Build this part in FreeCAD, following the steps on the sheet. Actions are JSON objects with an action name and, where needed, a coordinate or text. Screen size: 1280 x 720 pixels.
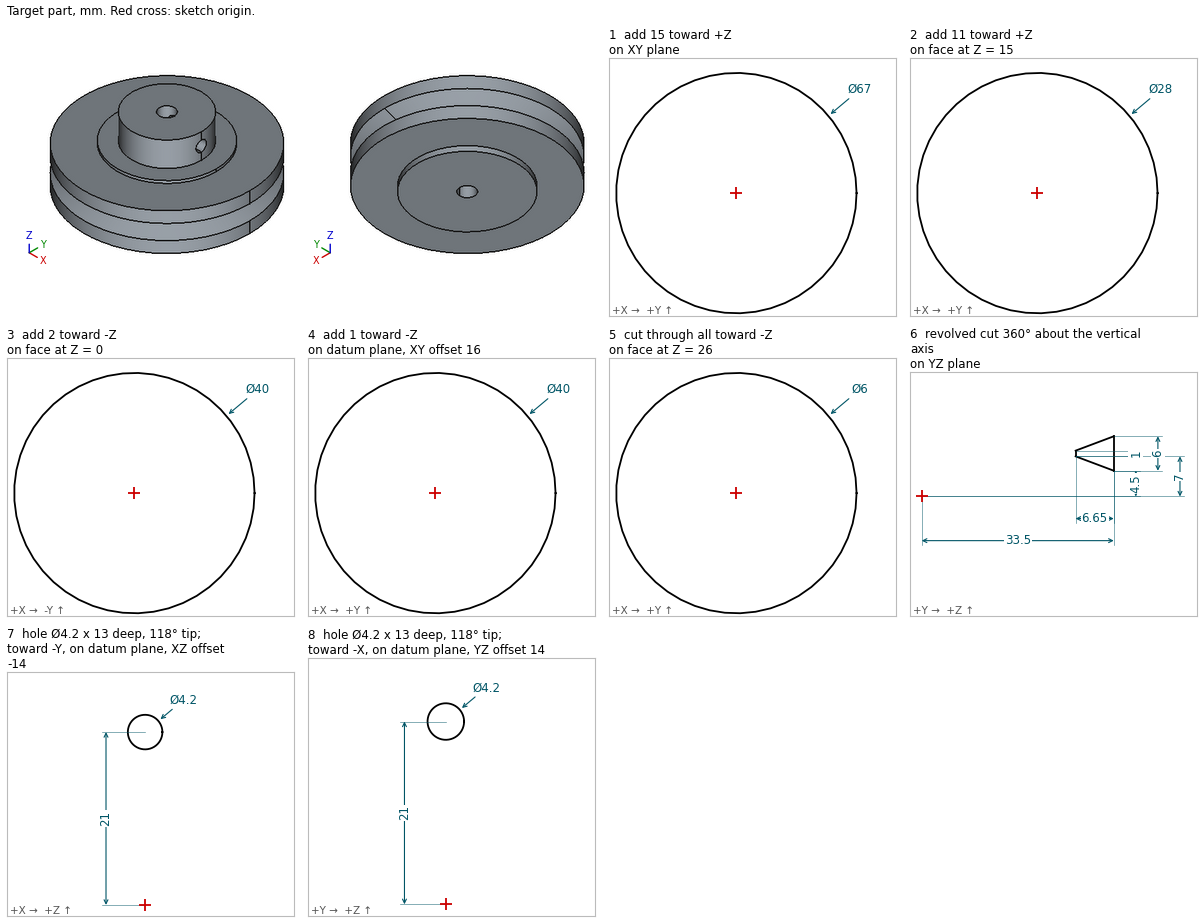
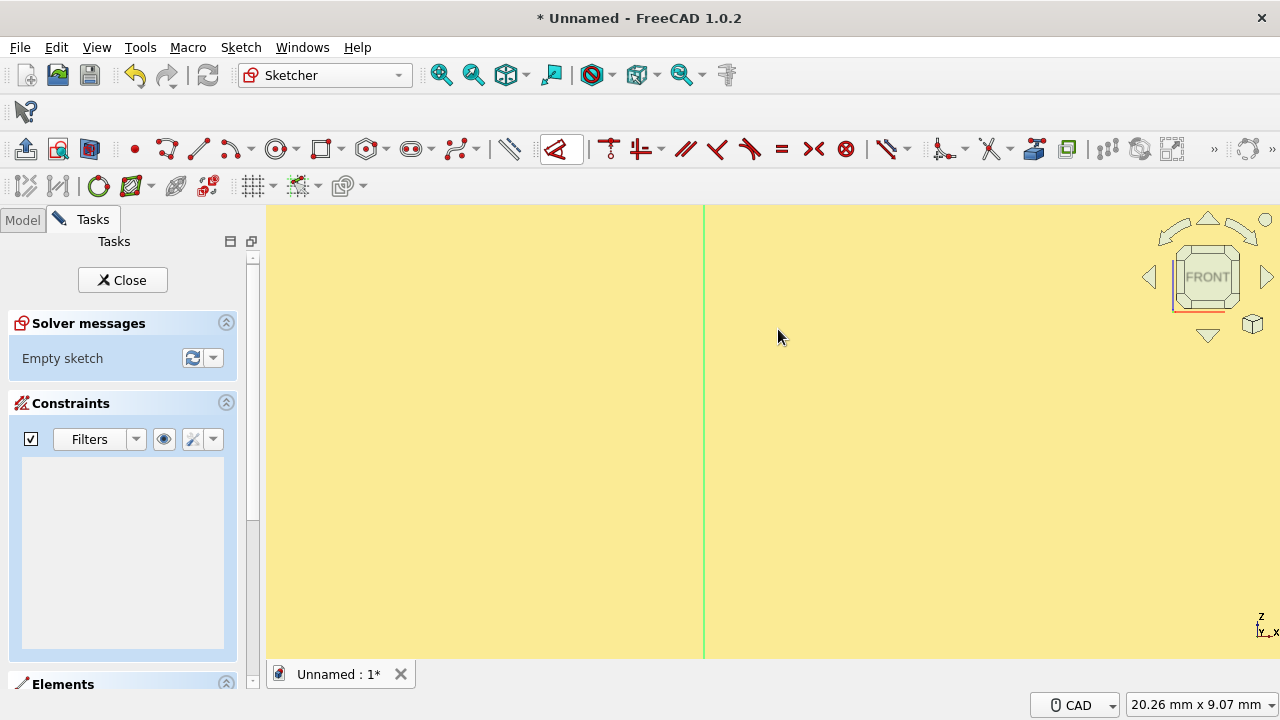
{"action": "left_click", "coordinate": [276, 150]}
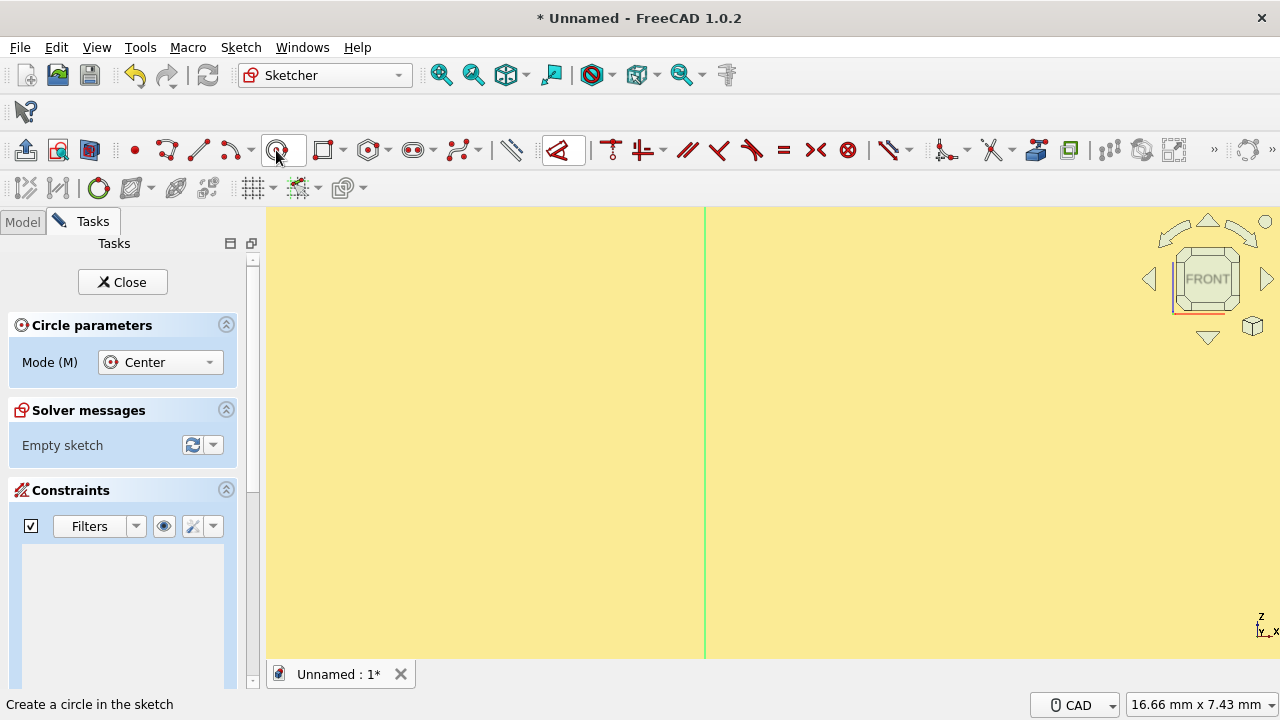
{"action": "left_click", "coordinate": [705, 430]}
{"action": "left_click", "coordinate": [795, 339]}
{"action": "key", "text": "Escape"}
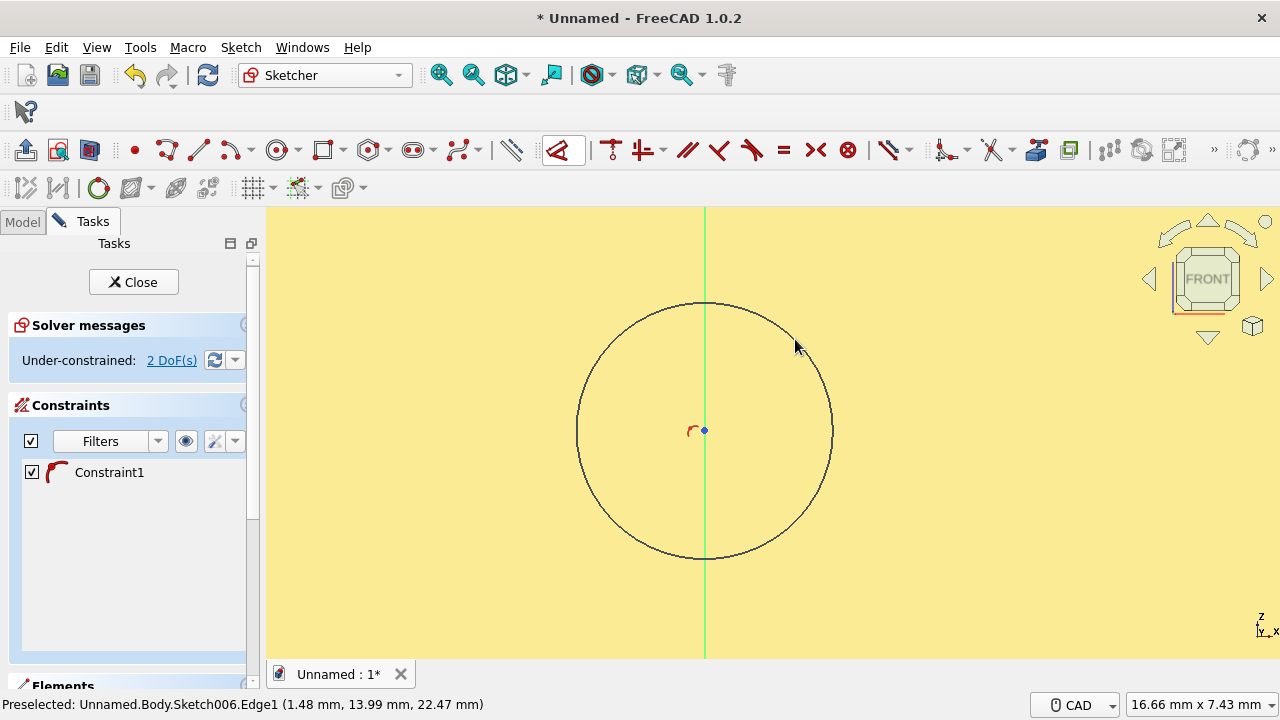
{"action": "left_click", "coordinate": [795, 340]}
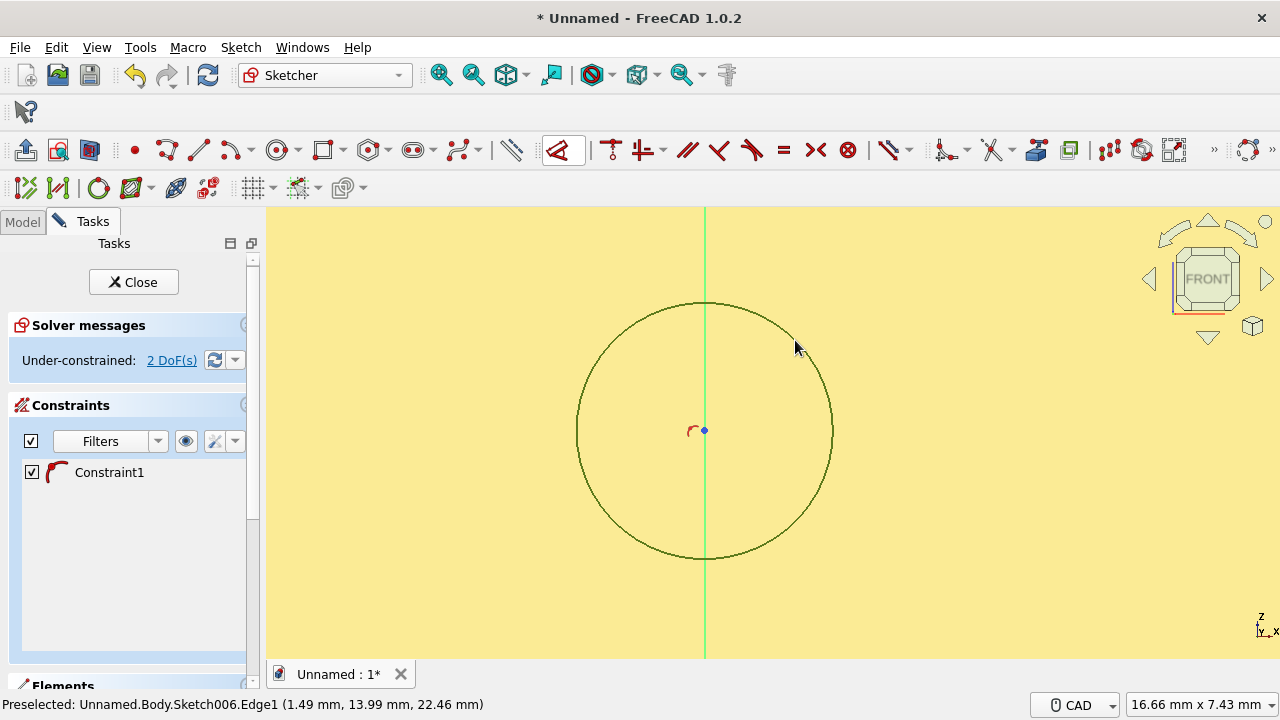
{"action": "key", "text": "k o"}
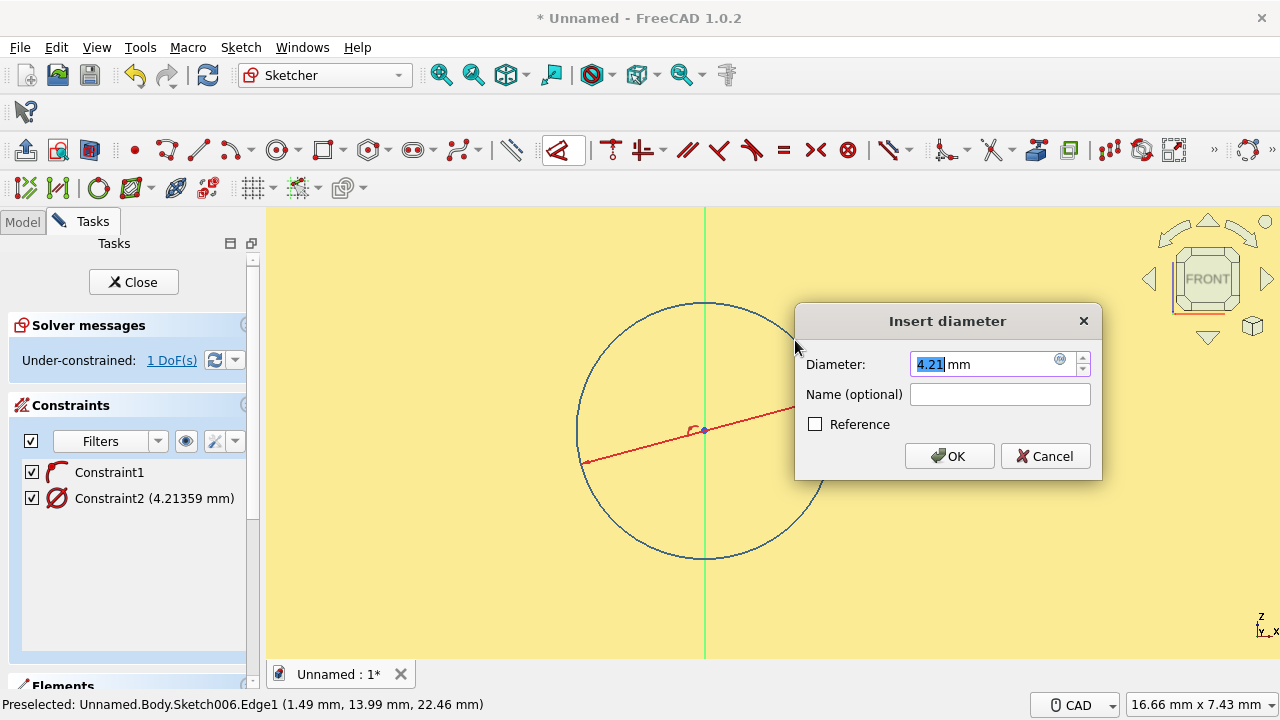
{"action": "type", "text": "4.2"}
{"action": "key", "text": "Return"}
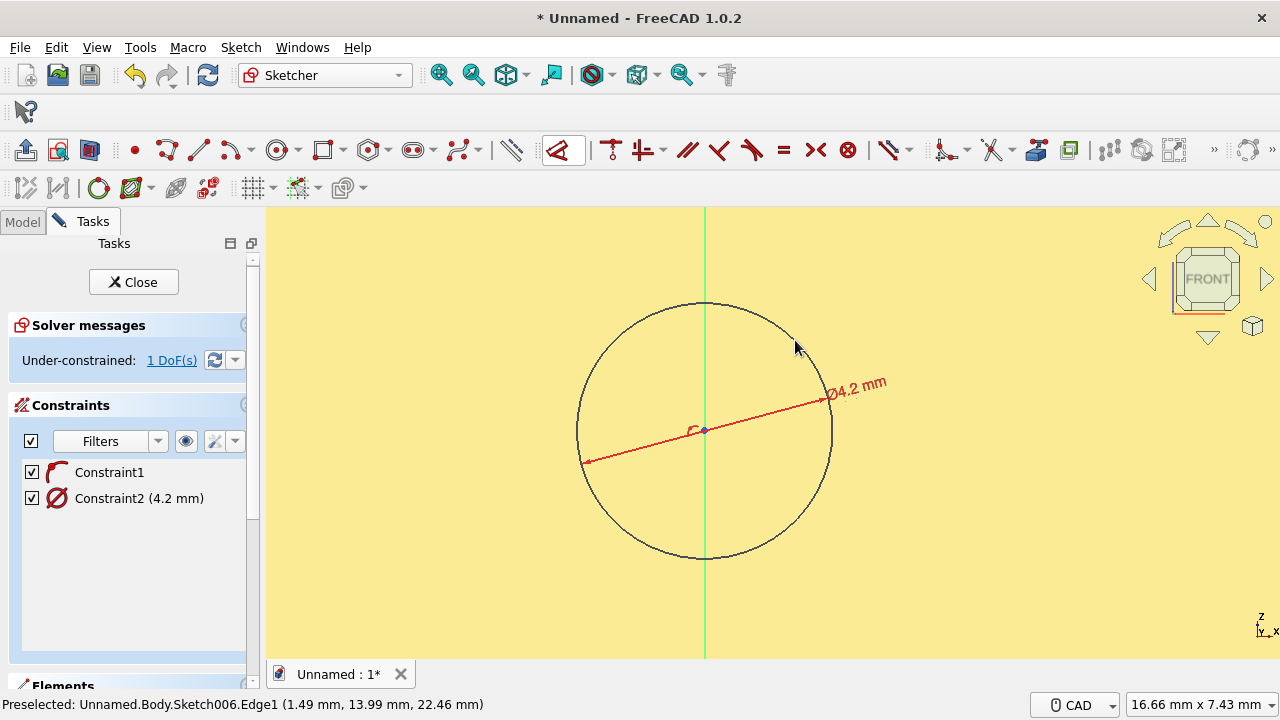
{"action": "left_click", "coordinate": [705, 431]}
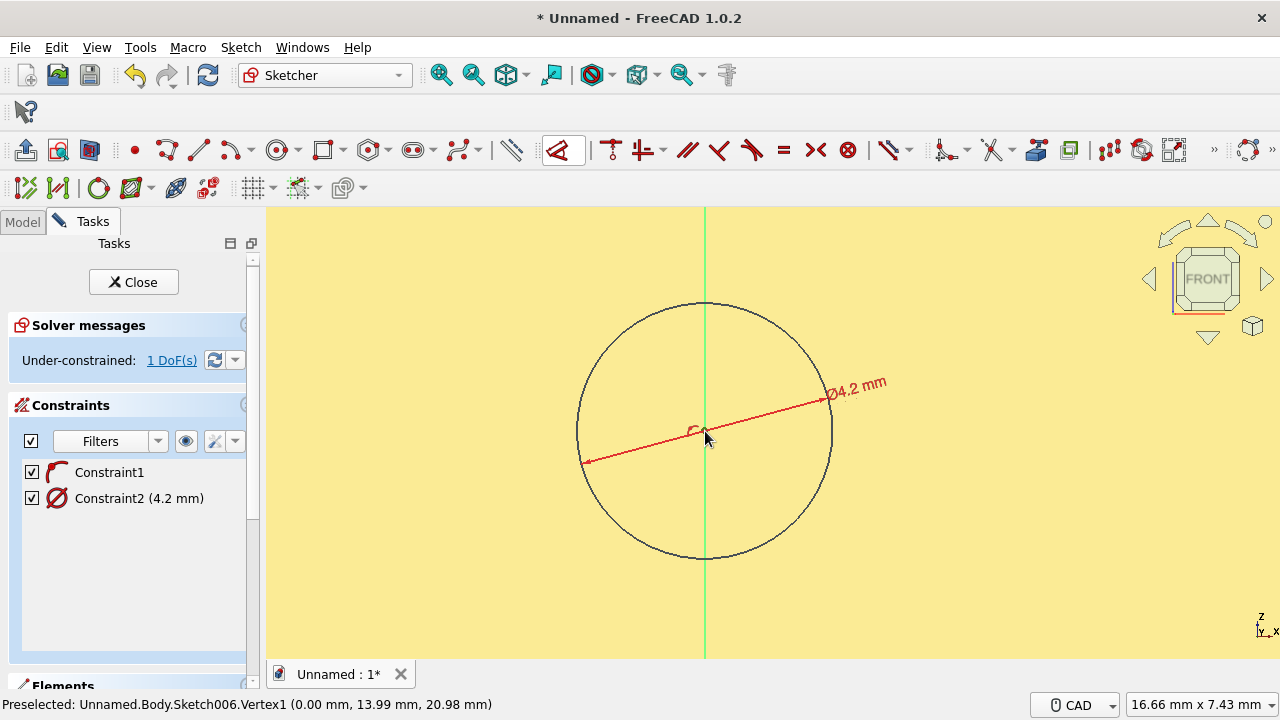
{"action": "key", "text": "i"}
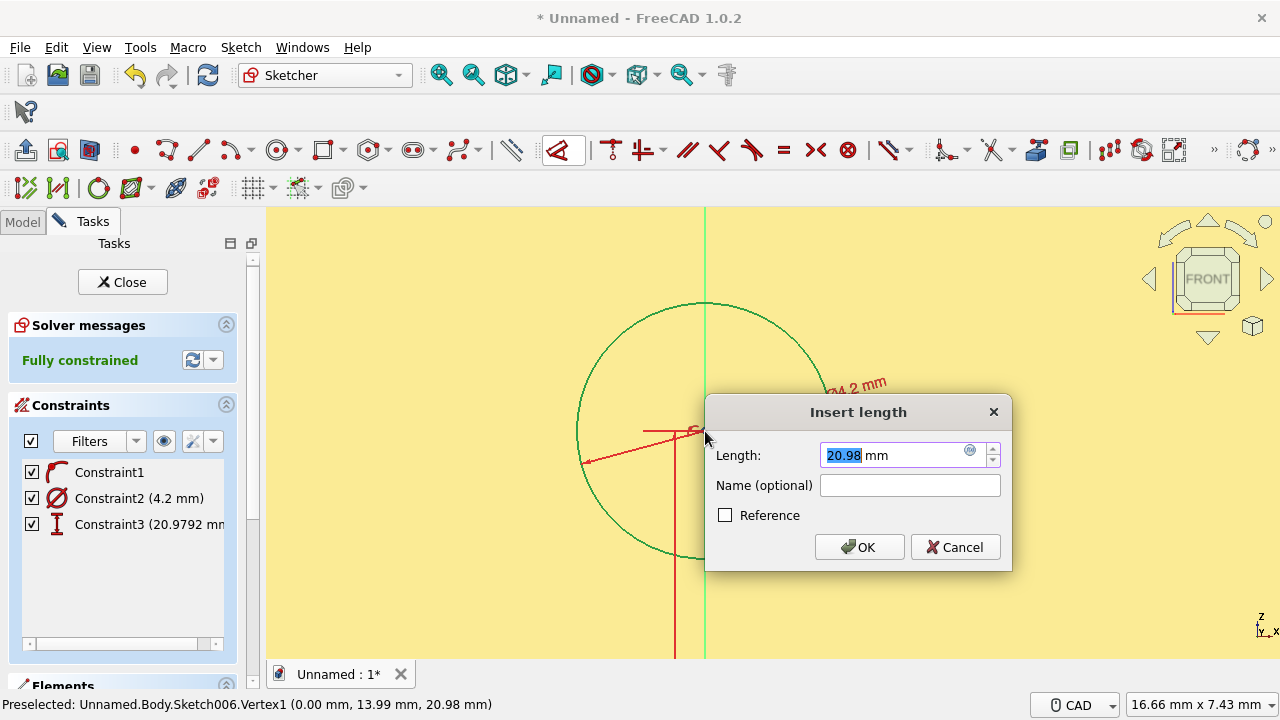
{"action": "type", "text": "21"}
{"action": "key", "text": "Return"}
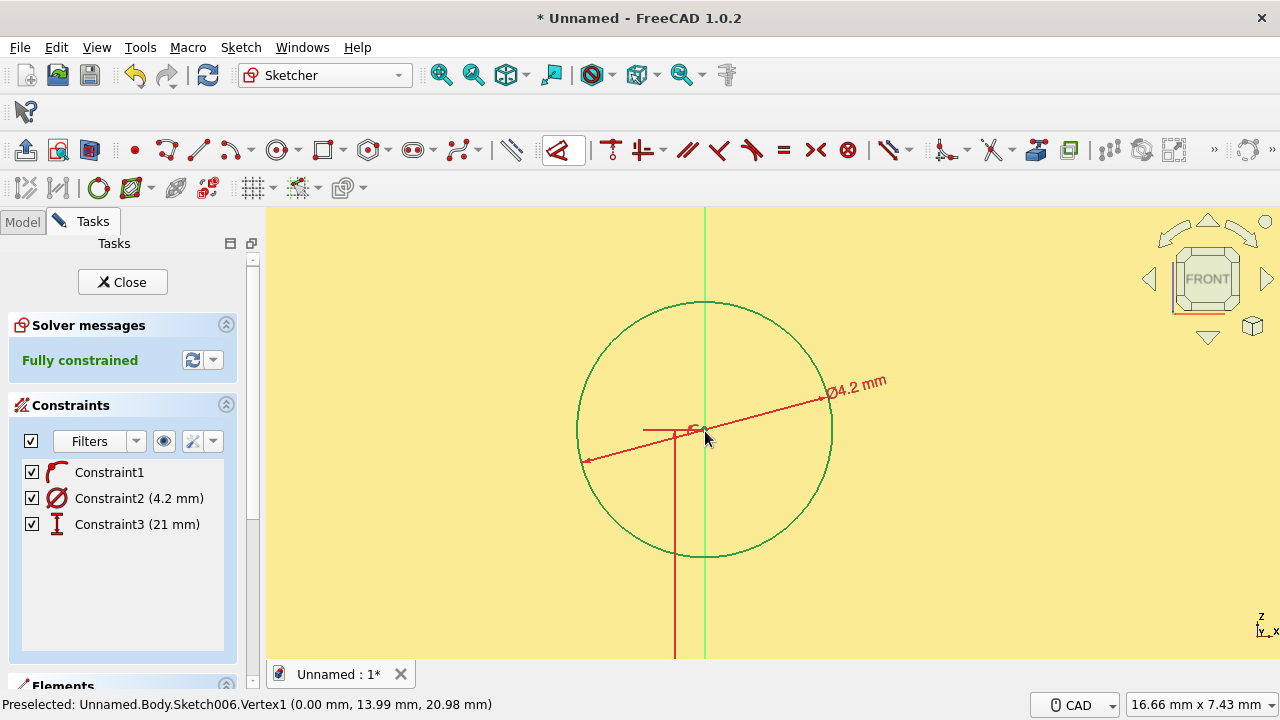
{"action": "left_click", "coordinate": [123, 282]}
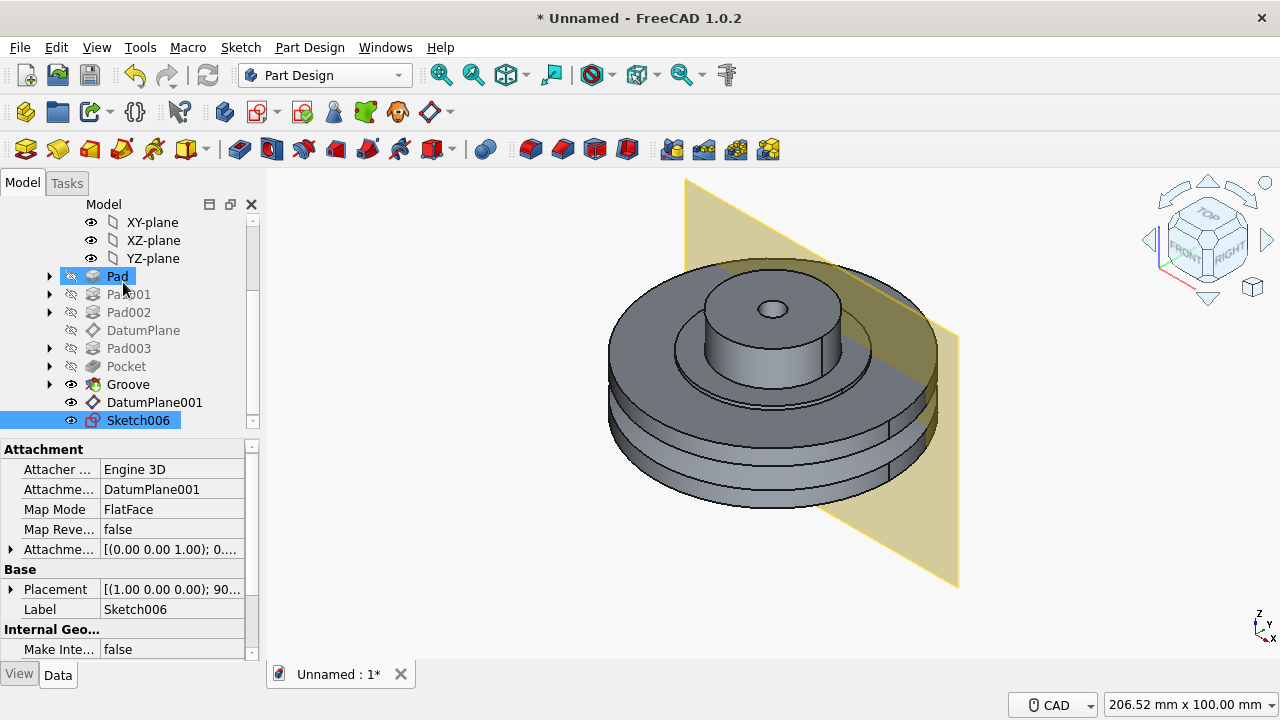
{"action": "left_click", "coordinate": [272, 150]}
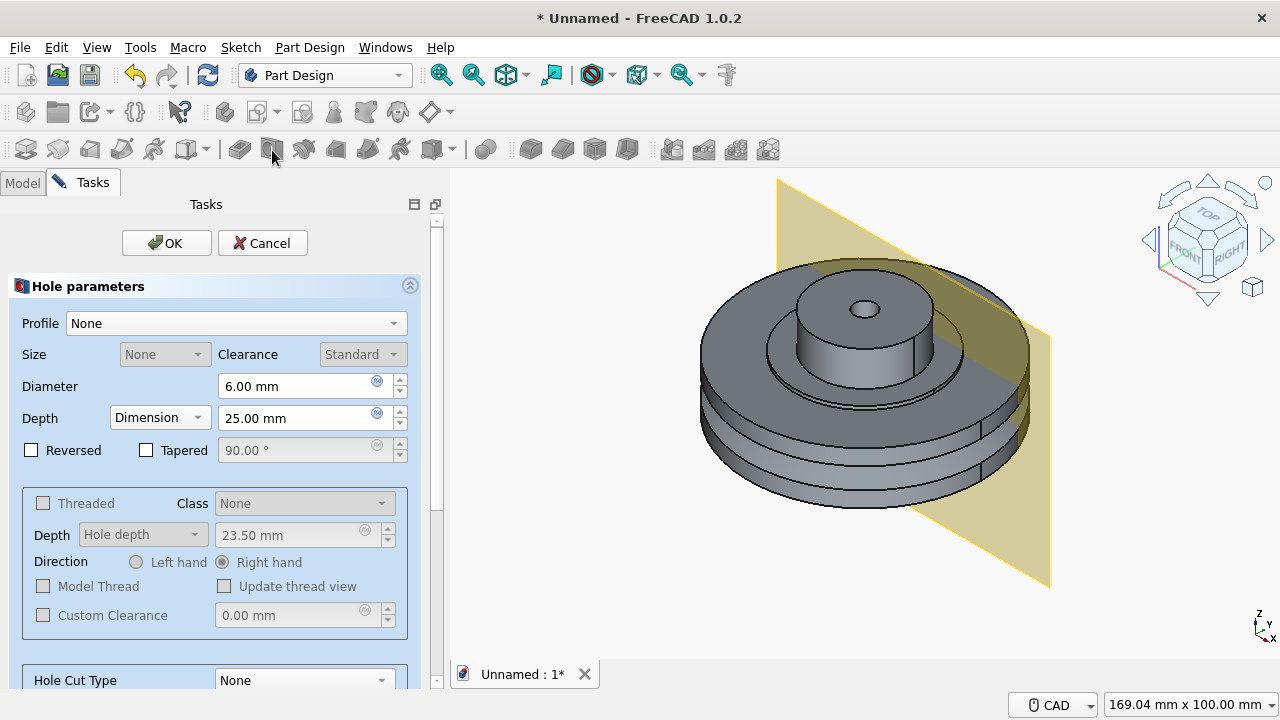
{"action": "triple_click", "coordinate": [305, 386]}